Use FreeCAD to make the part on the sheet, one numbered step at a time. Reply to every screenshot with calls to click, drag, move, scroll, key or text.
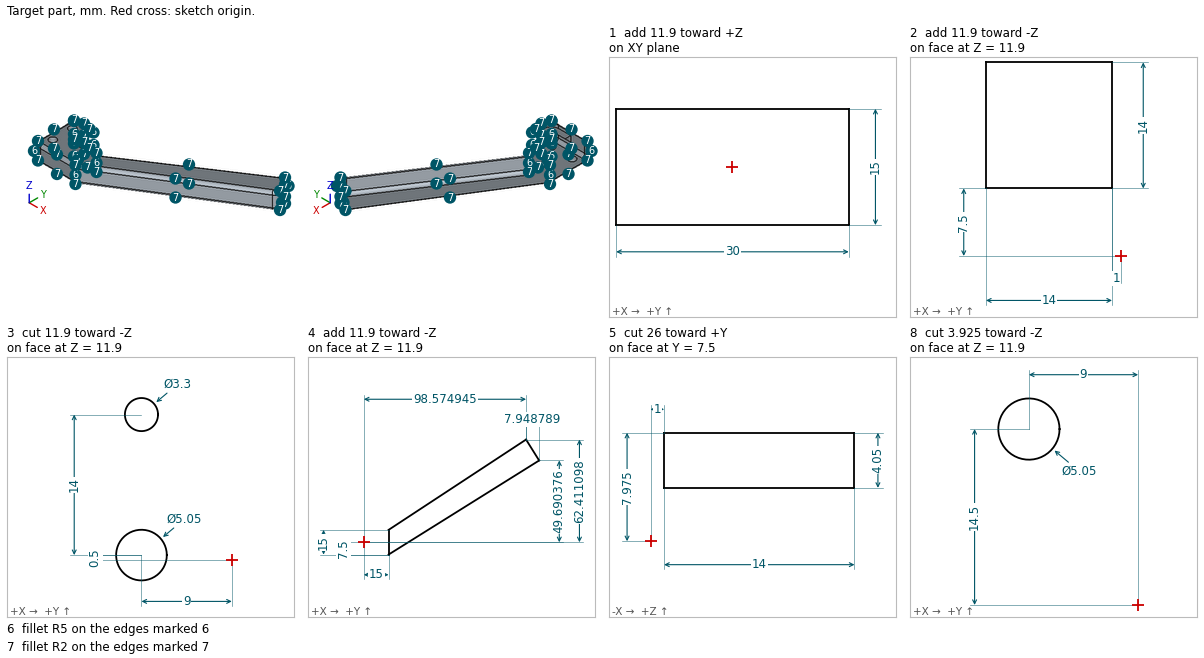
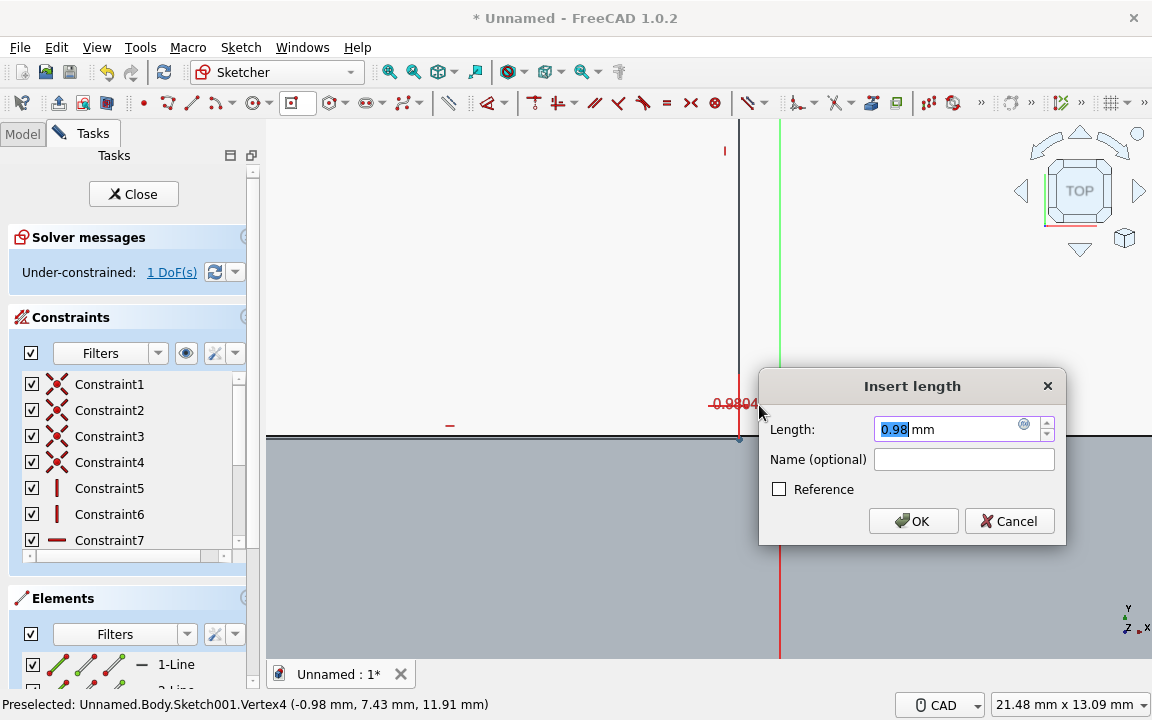
text(1)
key(Return)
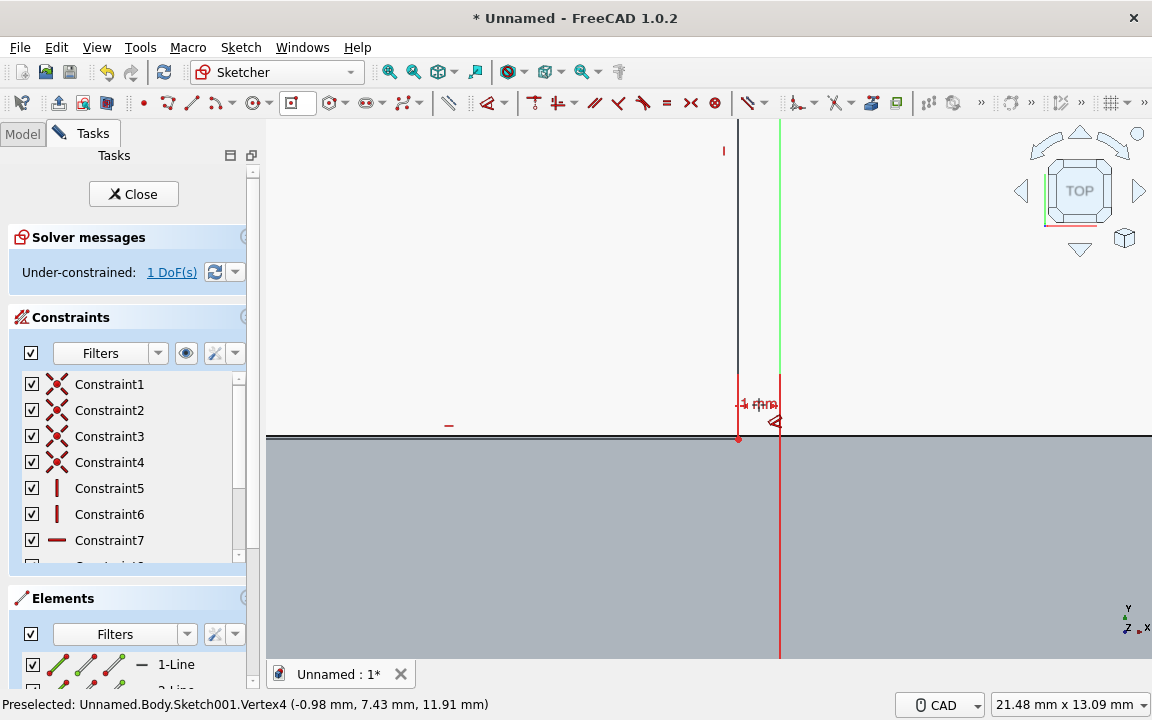
scroll(740, 440, down, 5)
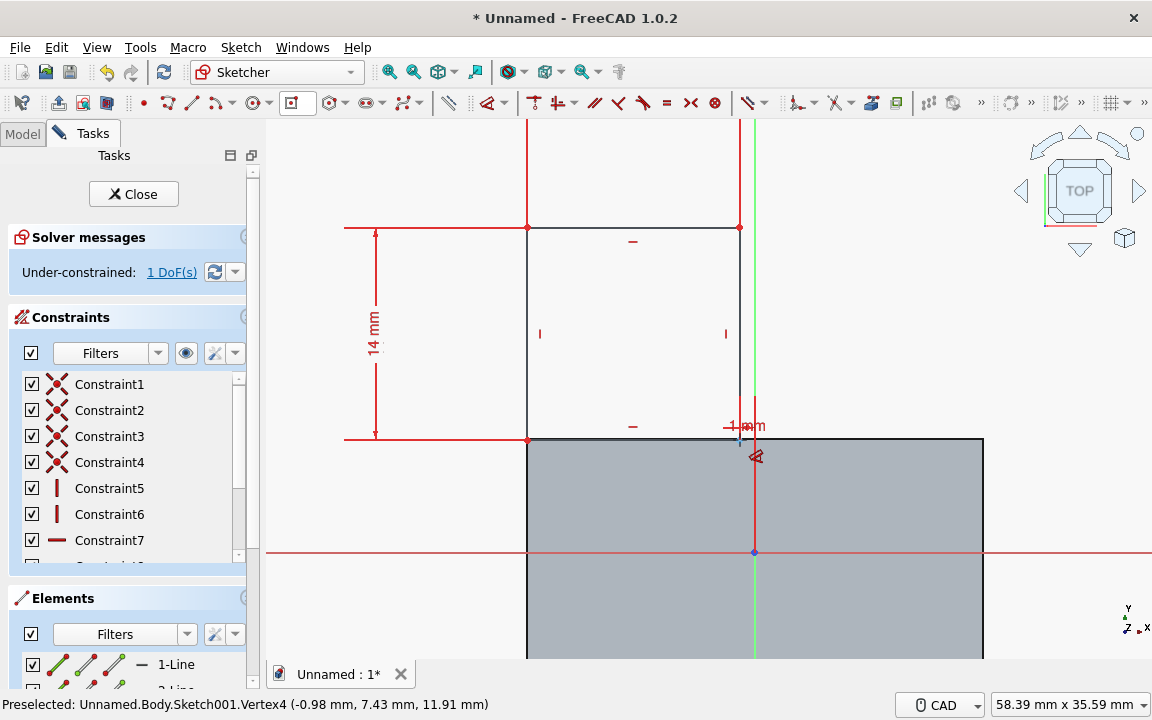
click(527, 440)
click(789, 496)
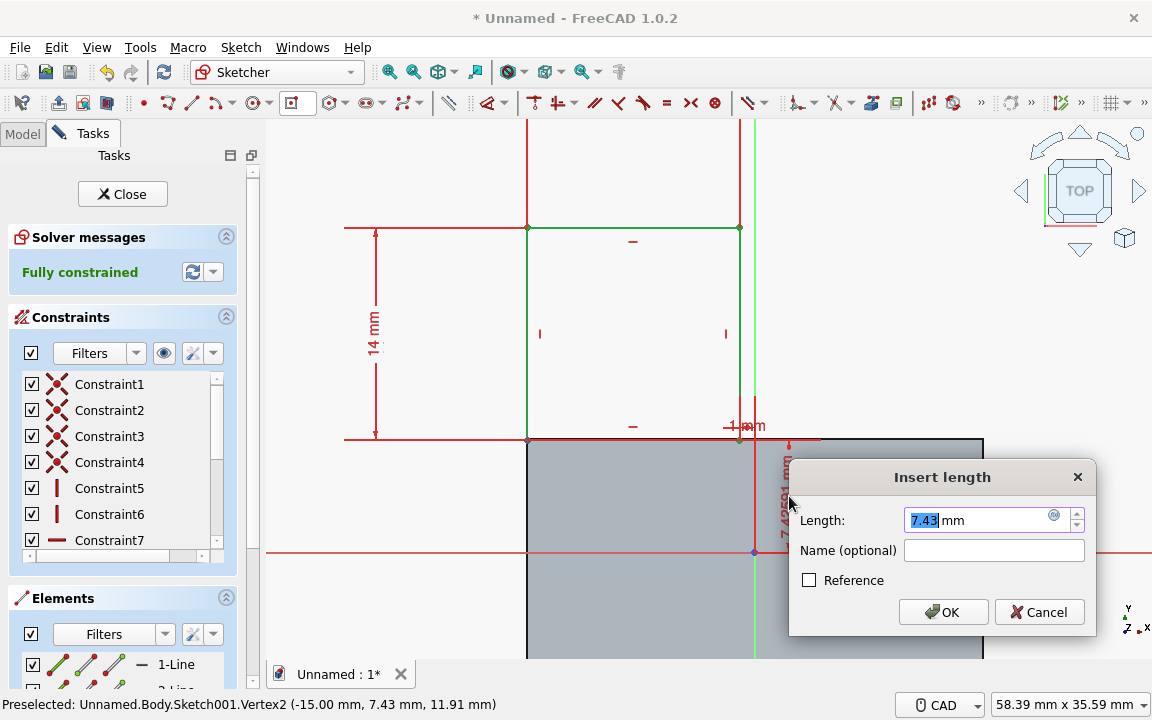
text(7.5)
key(Return)
key(Escape)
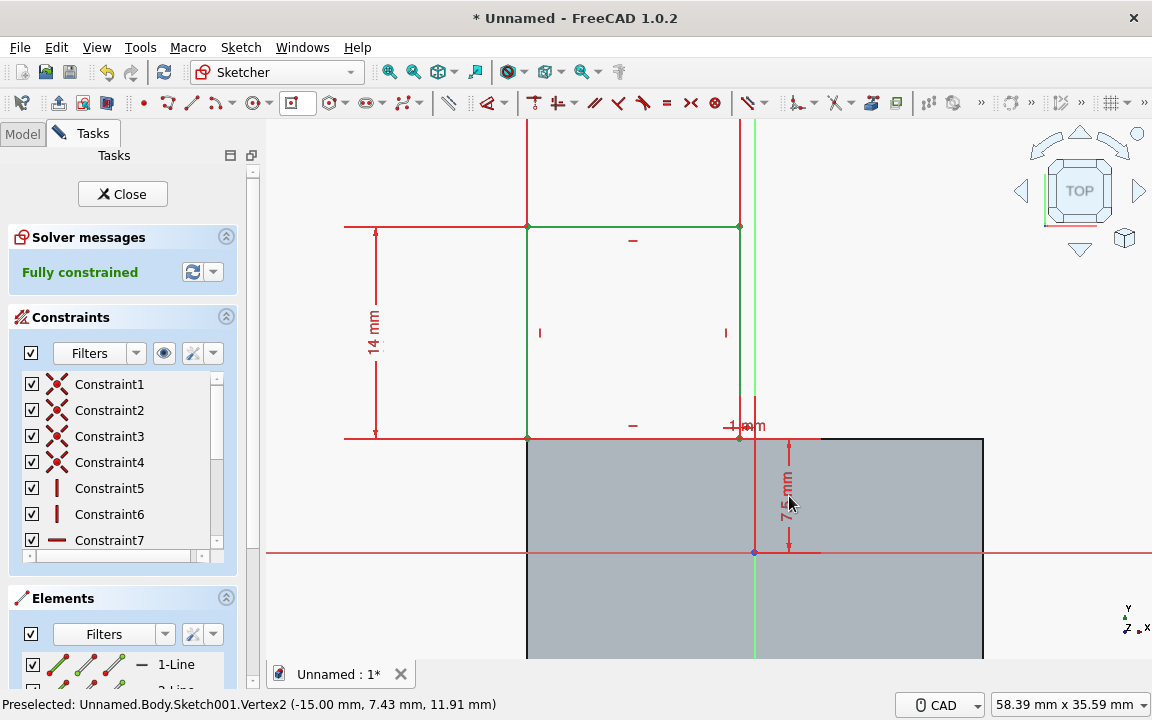
click(123, 194)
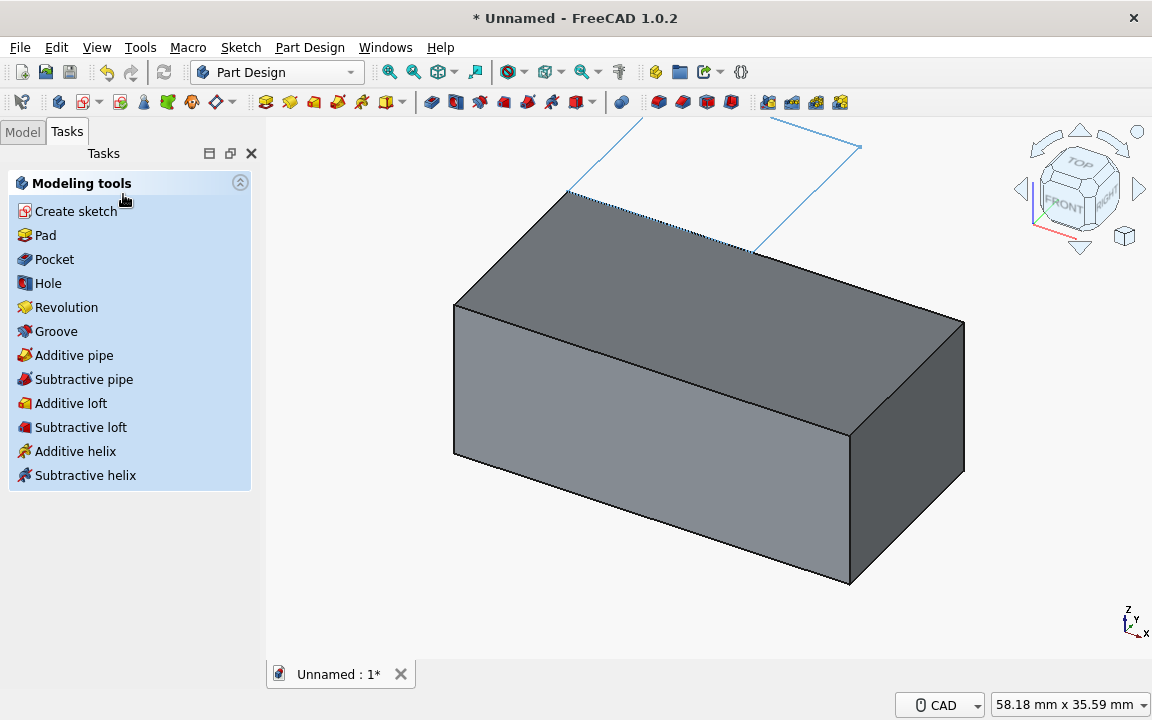
click(266, 102)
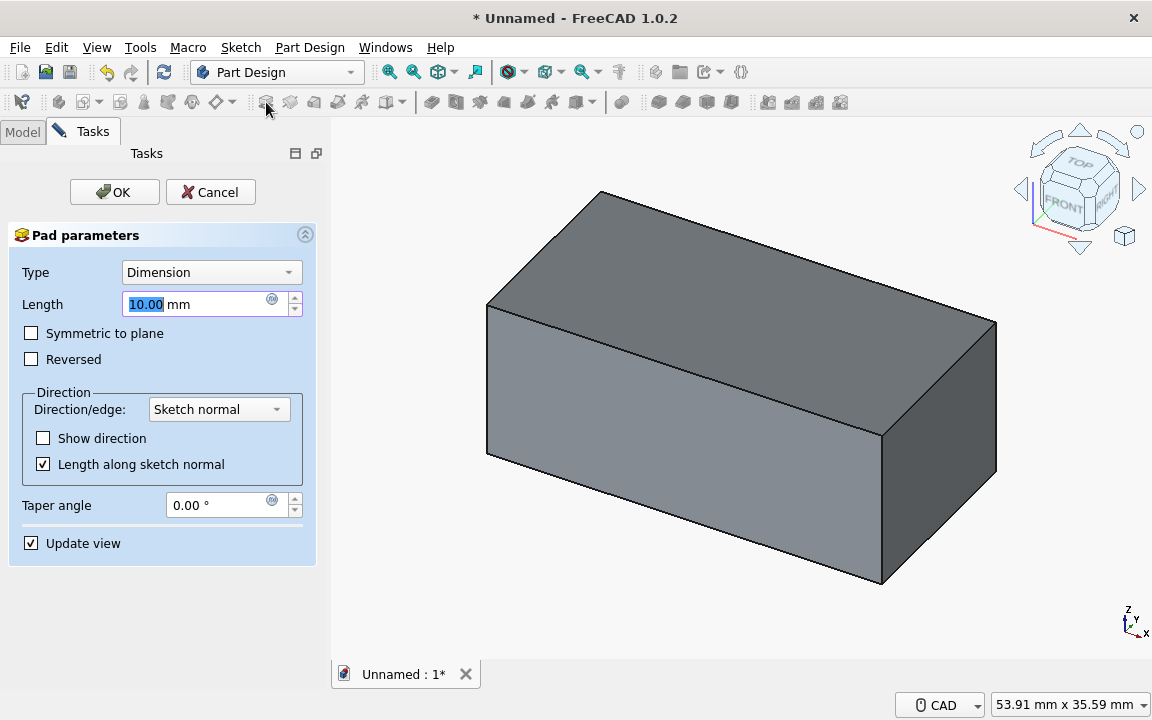
text(11.9)
key(Tab)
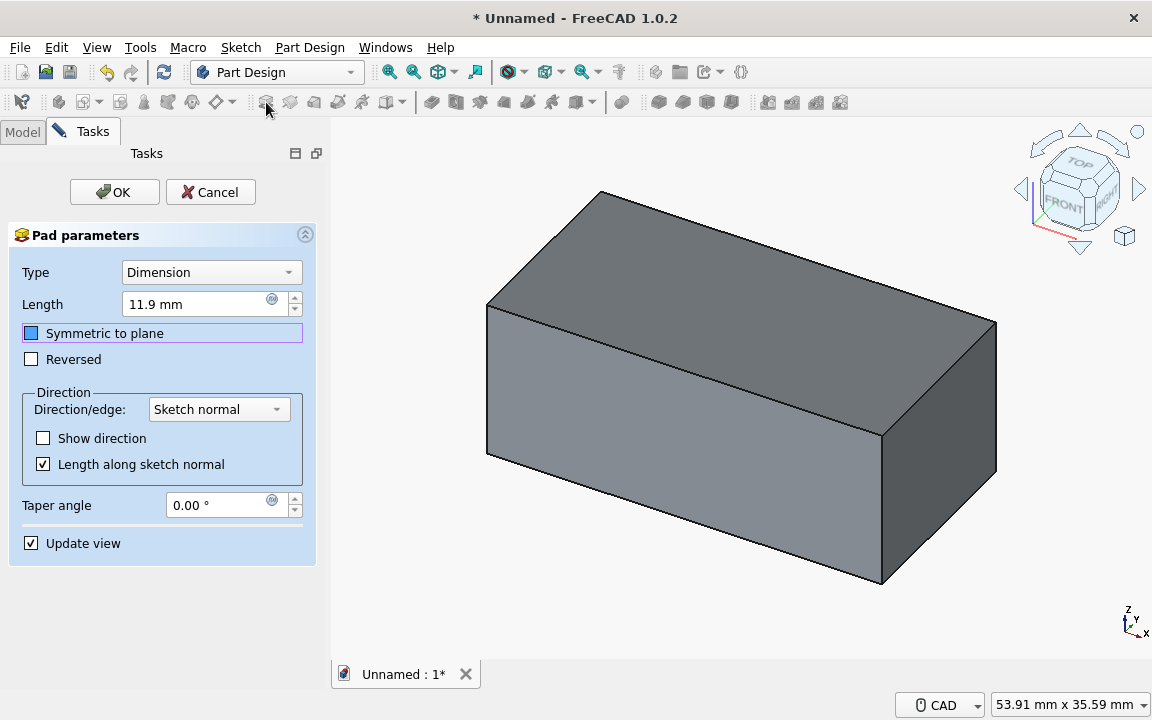
click(30, 359)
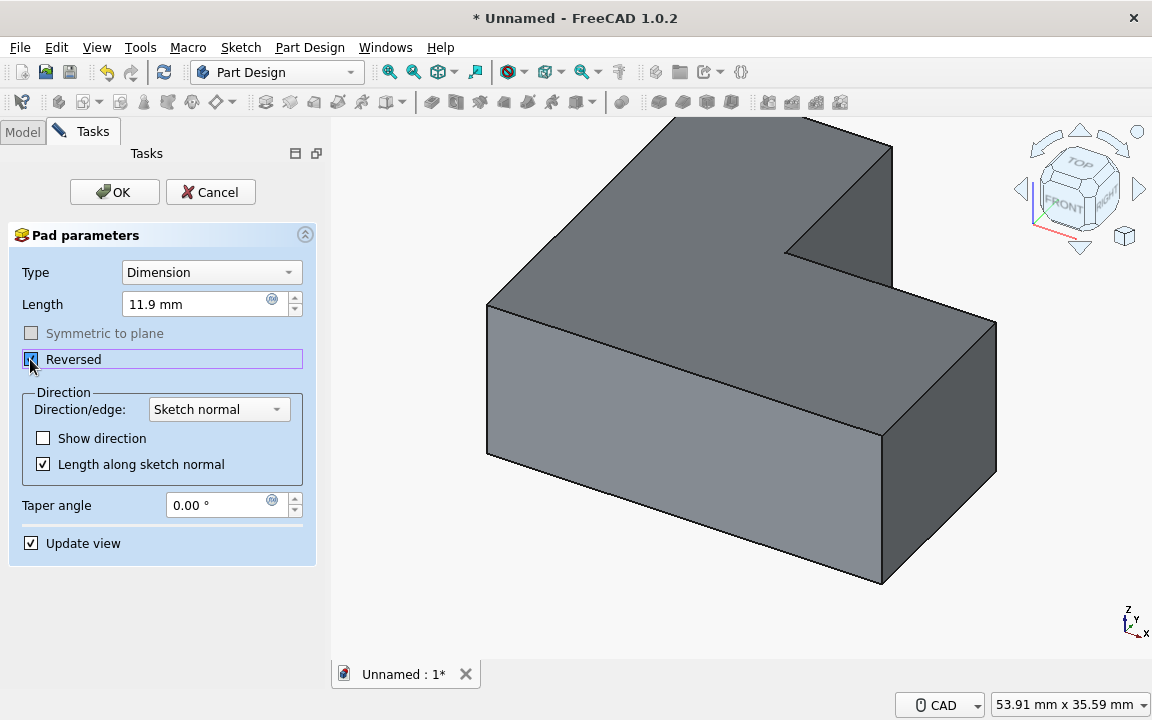
click(115, 192)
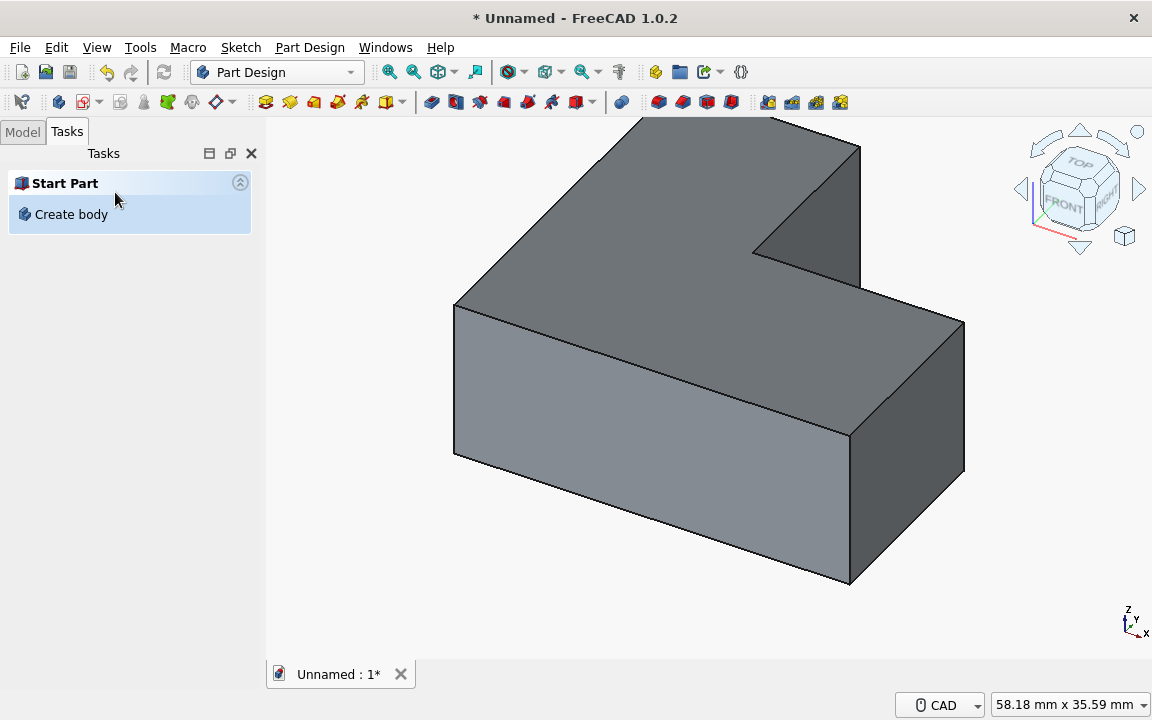
click(390, 72)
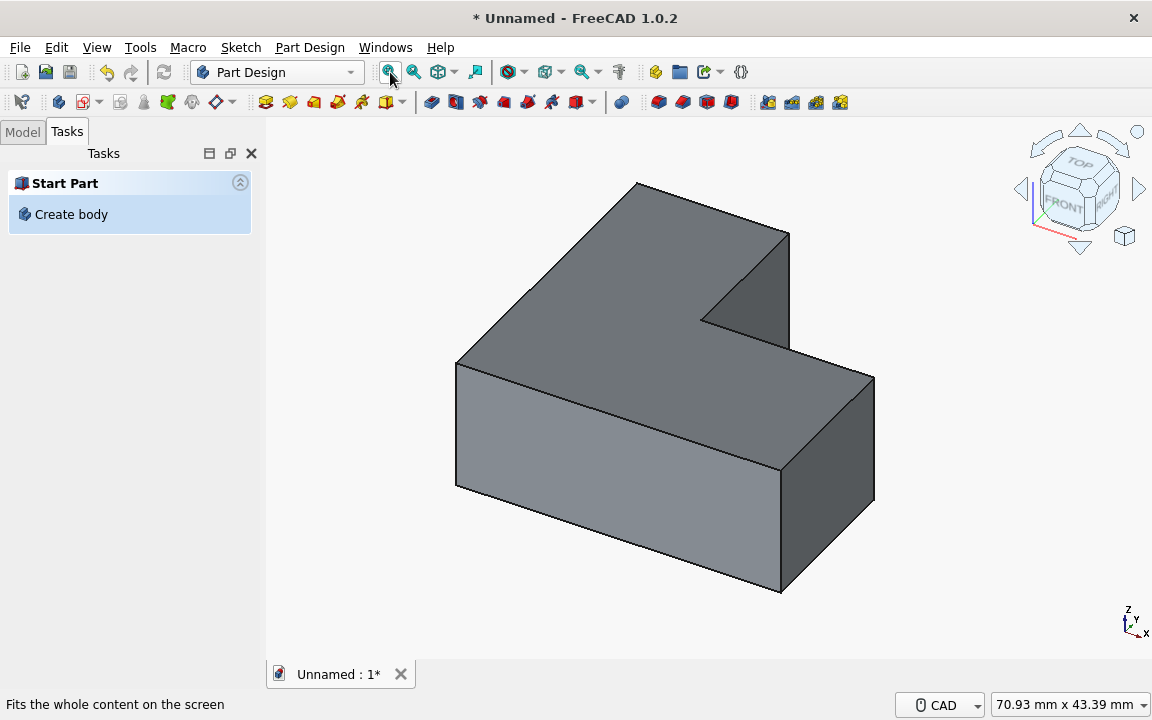
click(642, 270)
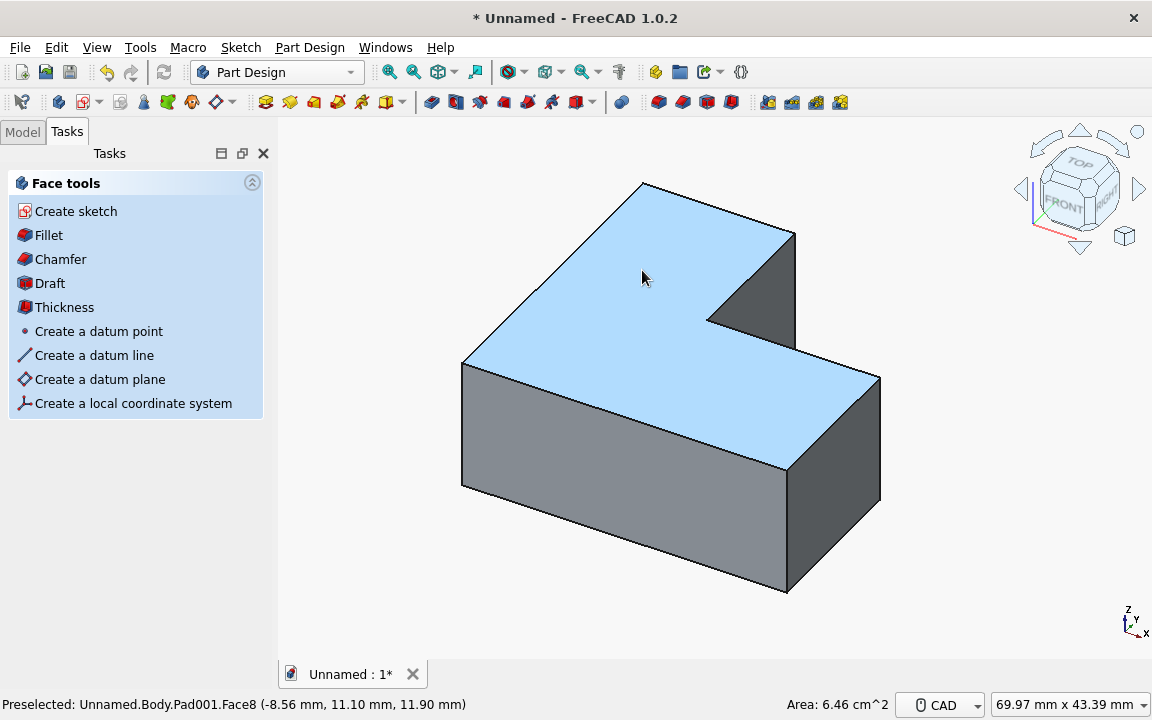
click(84, 102)